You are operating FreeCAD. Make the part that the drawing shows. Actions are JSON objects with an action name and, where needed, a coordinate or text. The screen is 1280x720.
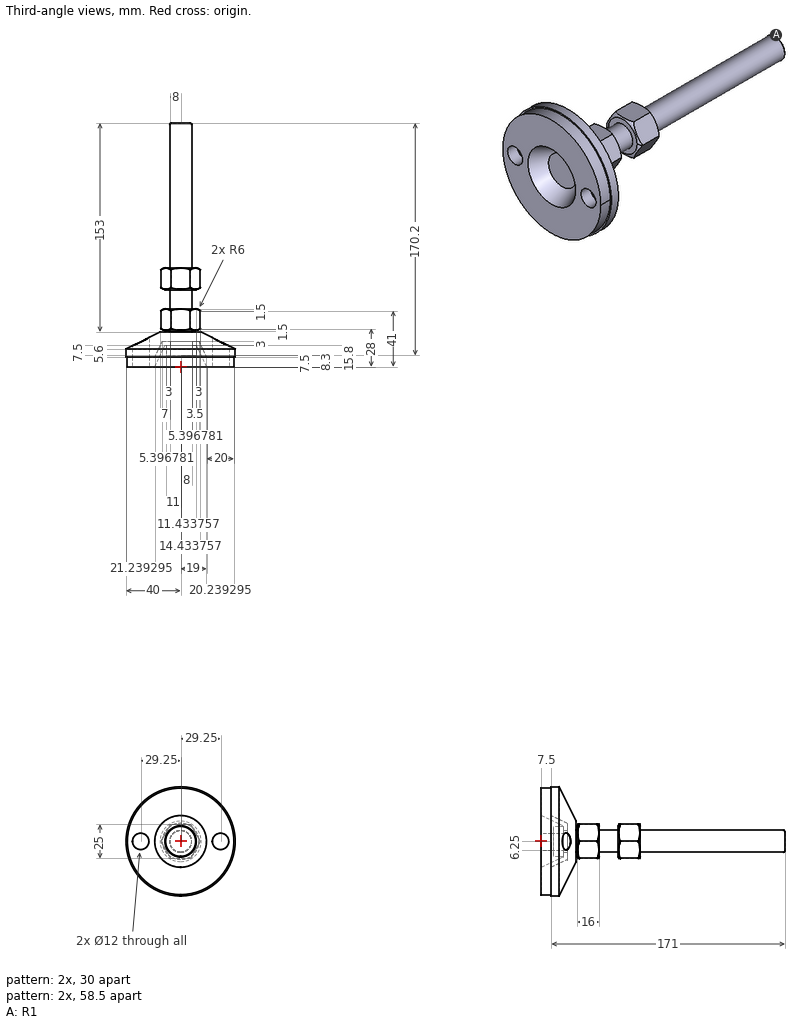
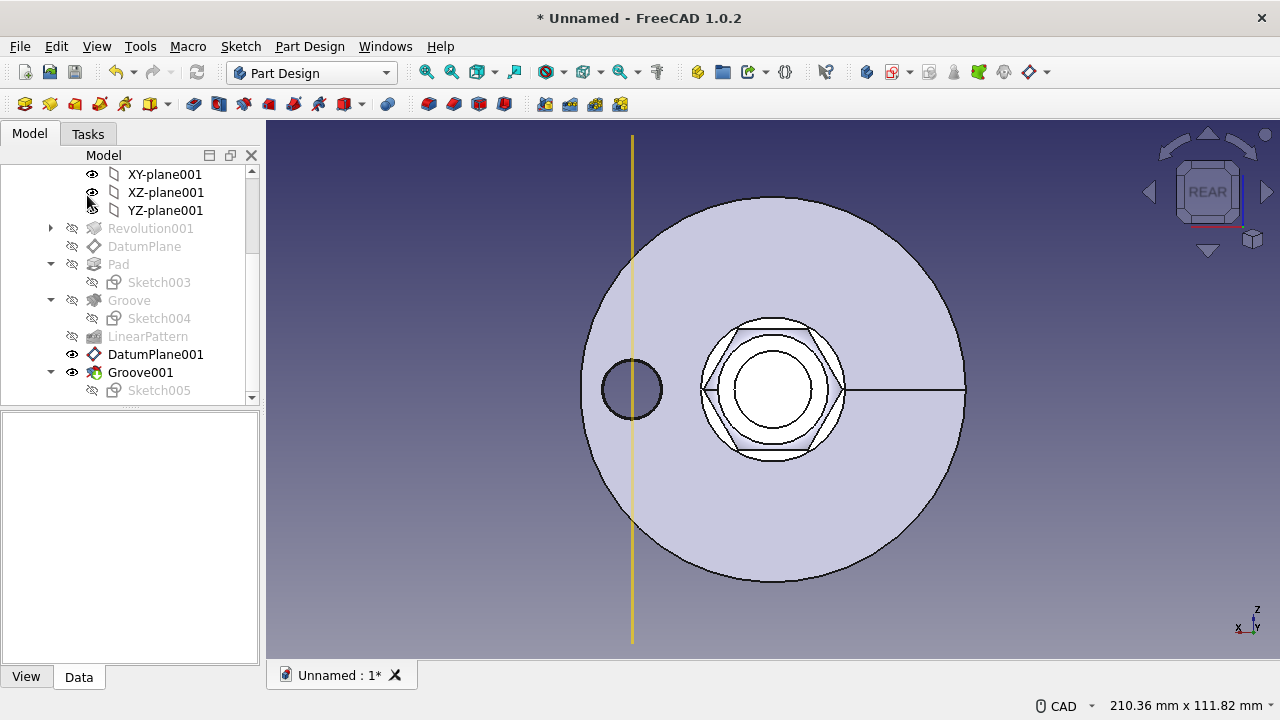
{"action": "left_click", "coordinate": [117, 354]}
{"action": "key", "text": "space"}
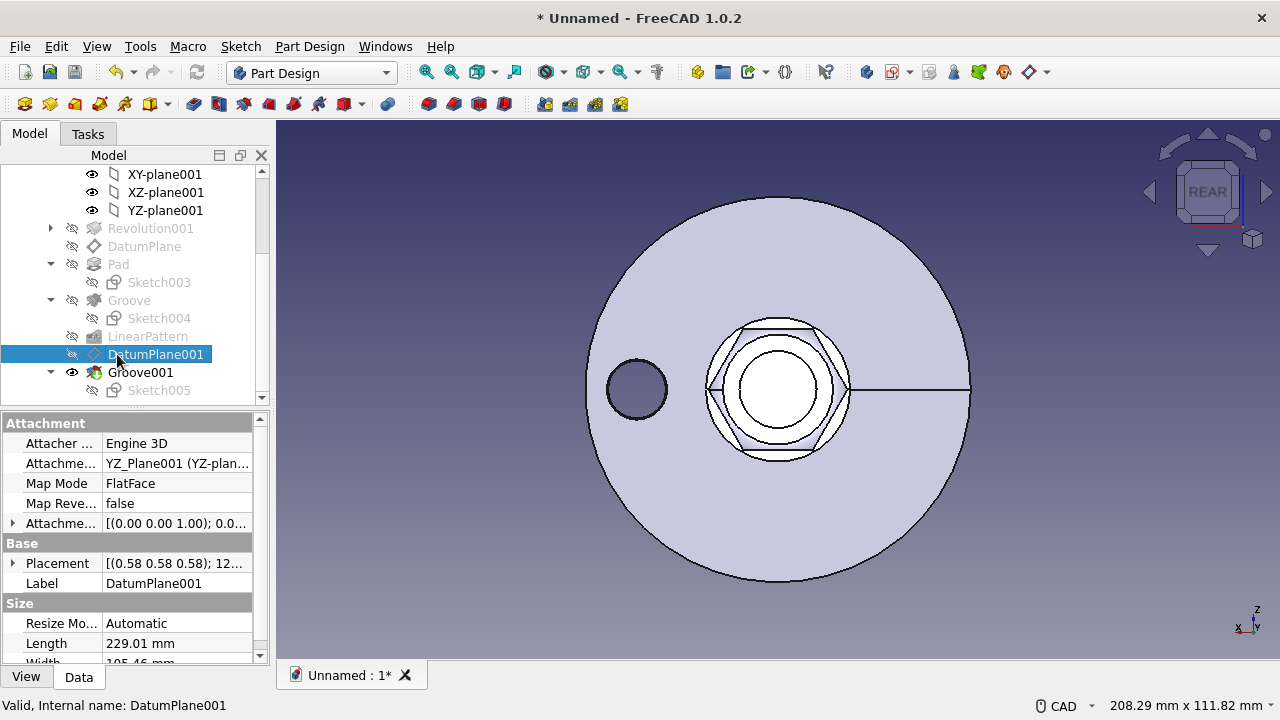
{"action": "left_click", "coordinate": [117, 372]}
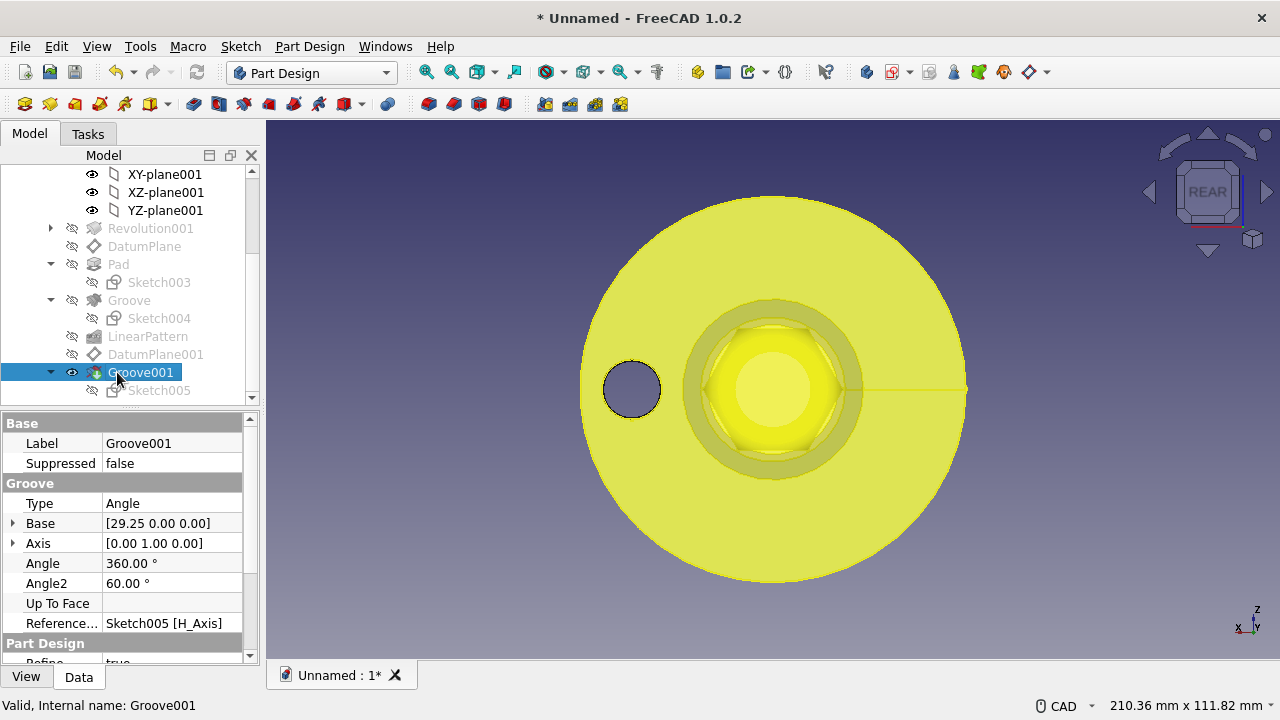
{"action": "left_click", "coordinate": [570, 104]}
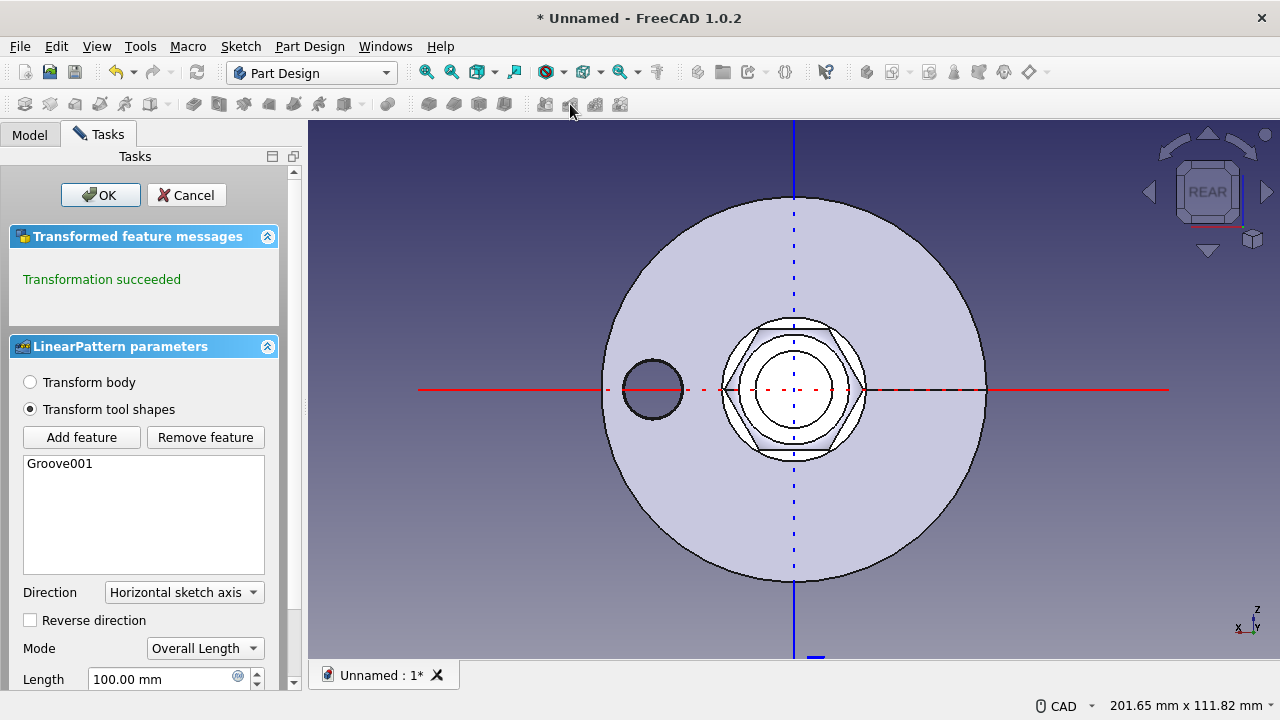
{"action": "left_click", "coordinate": [185, 592]}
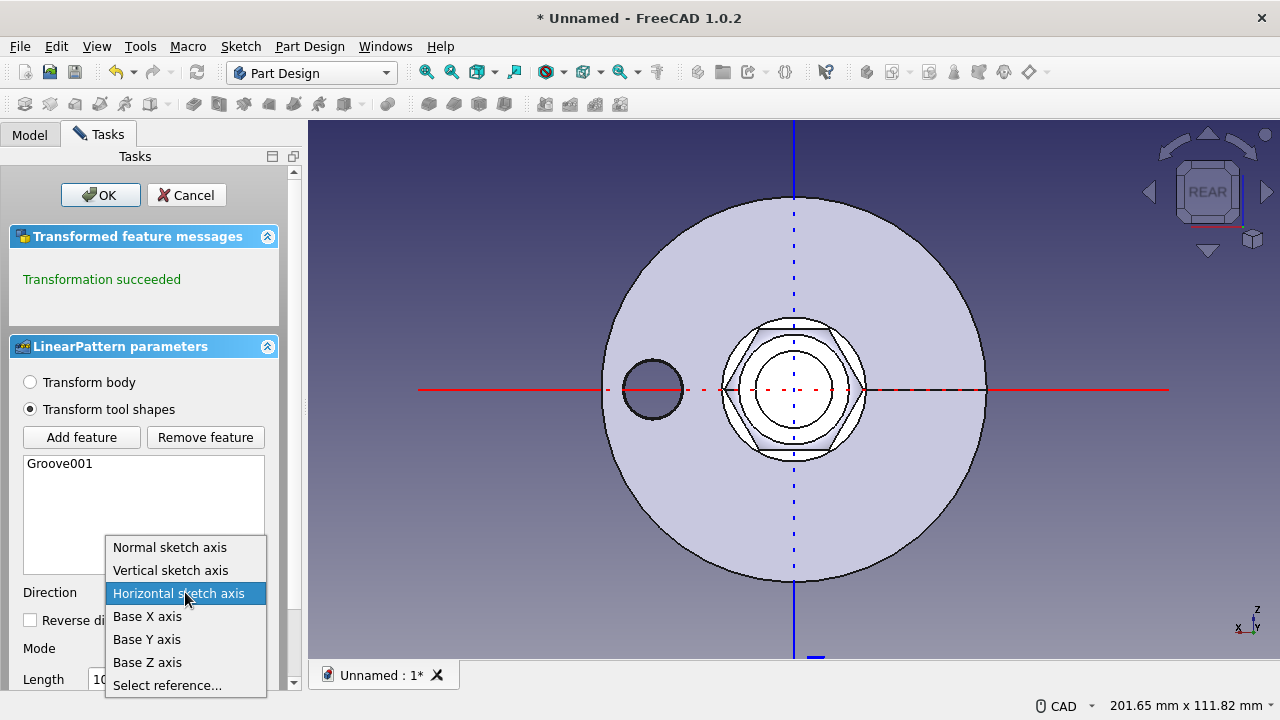
{"action": "left_click", "coordinate": [184, 616]}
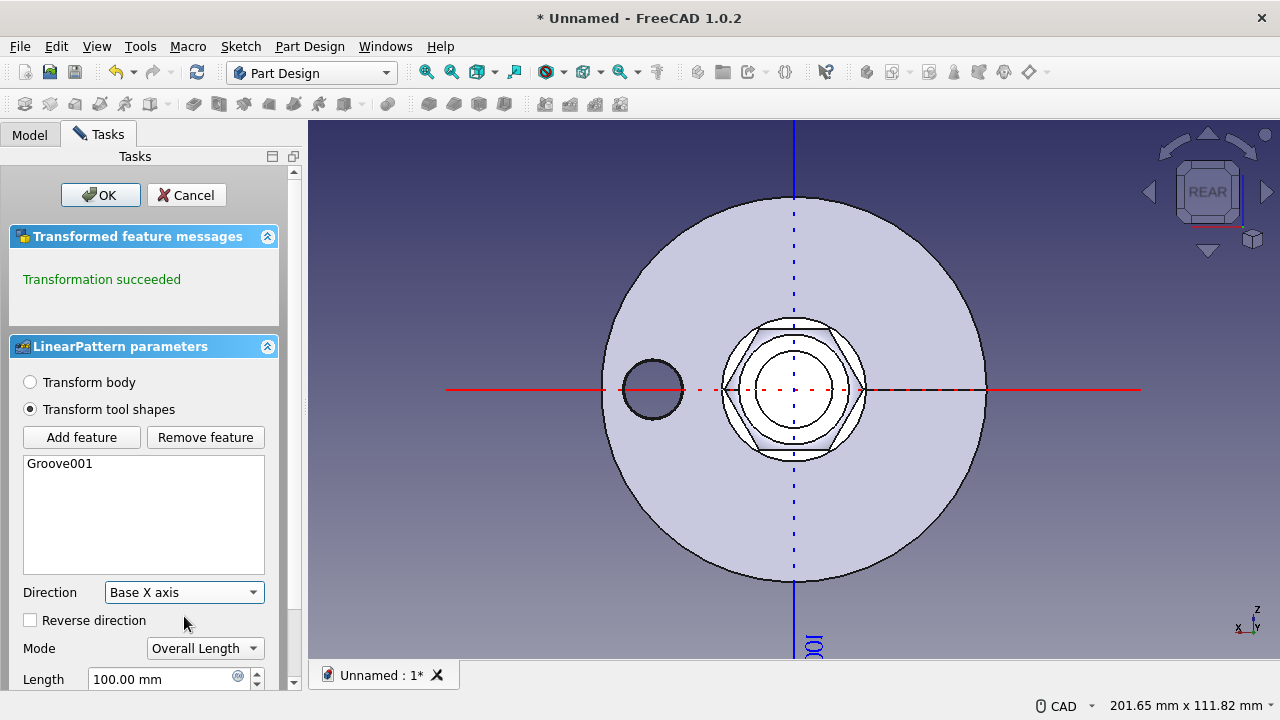
{"action": "left_click", "coordinate": [206, 648]}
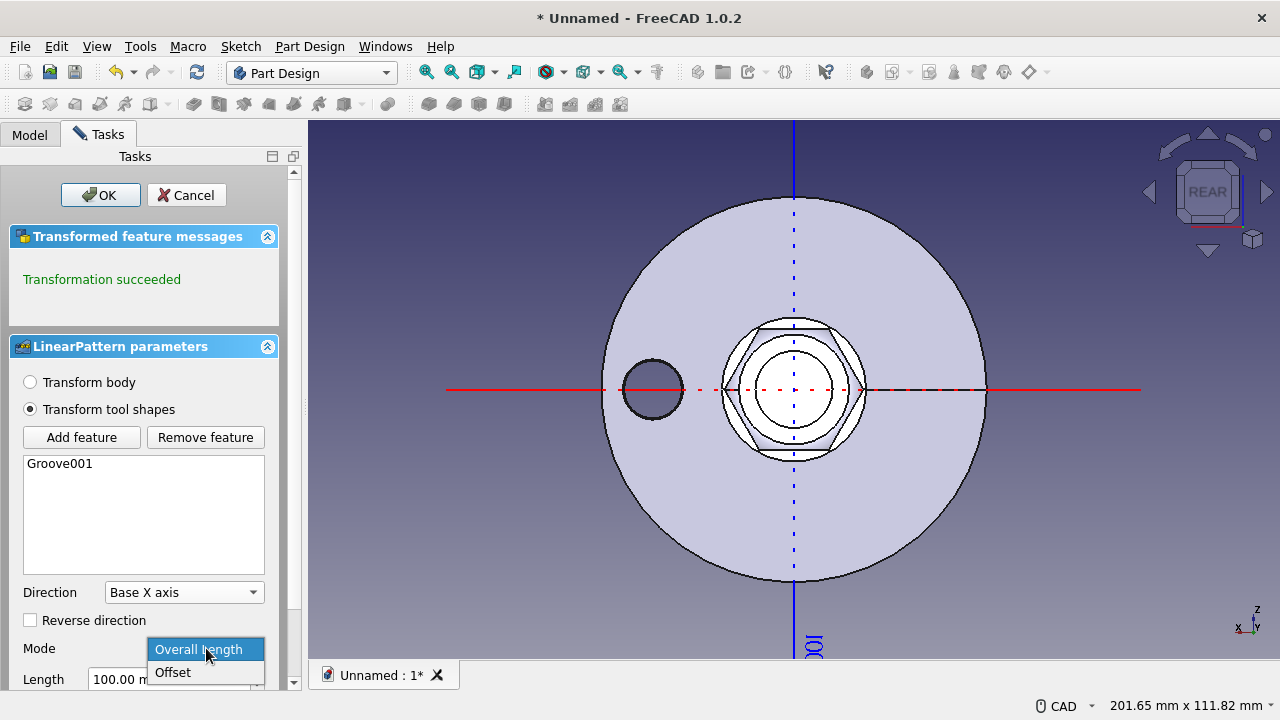
{"action": "left_click", "coordinate": [204, 672]}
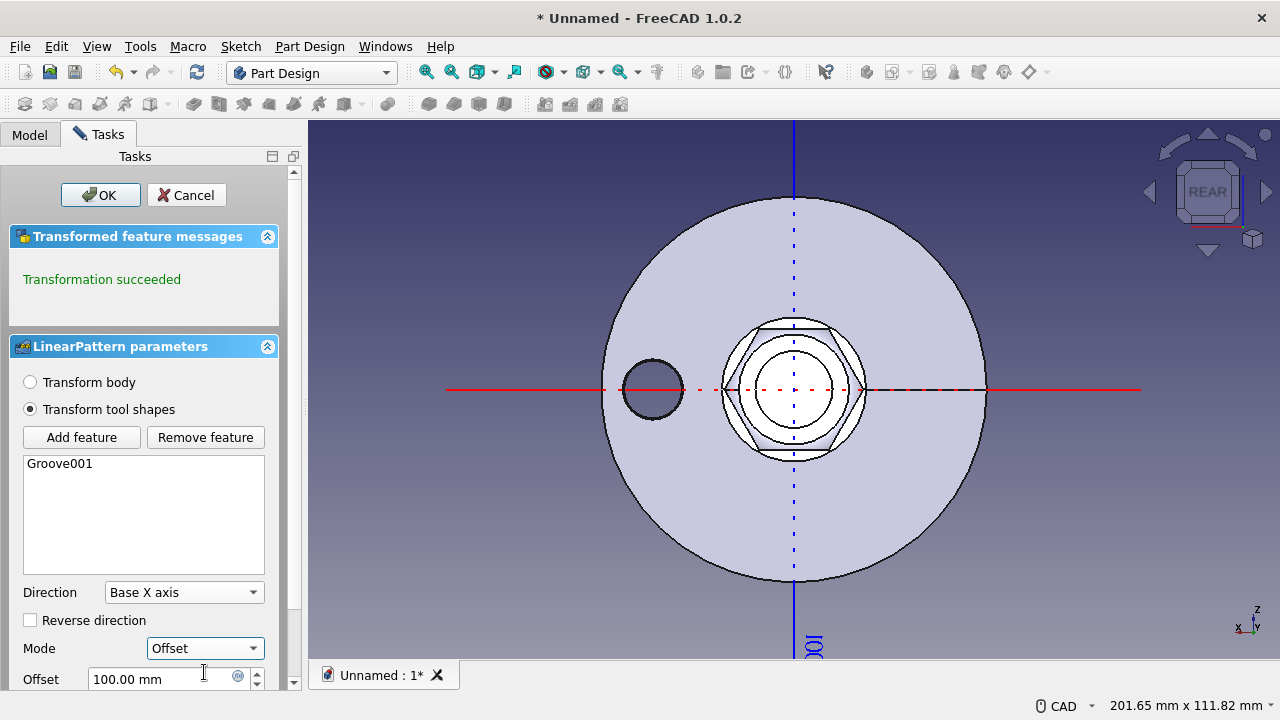
{"action": "scroll", "coordinate": [294, 428], "scroll_direction": "down", "scroll_amount": 2}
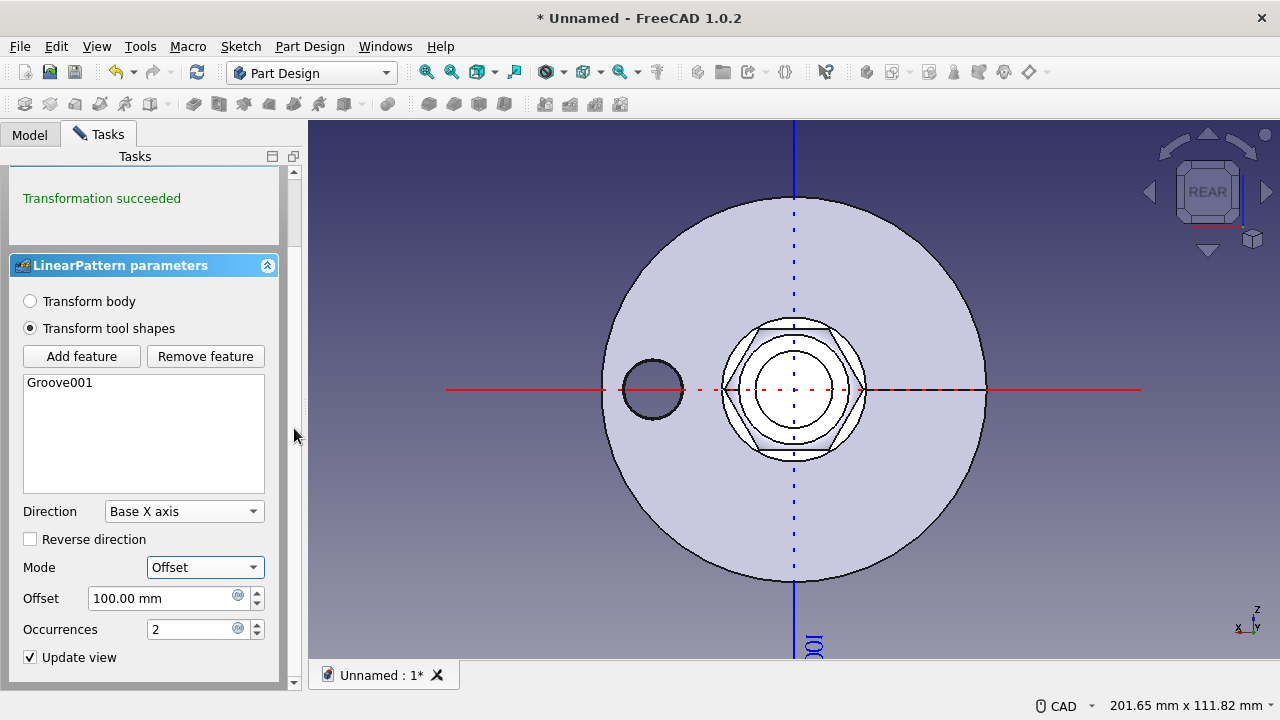
{"action": "triple_click", "coordinate": [170, 598]}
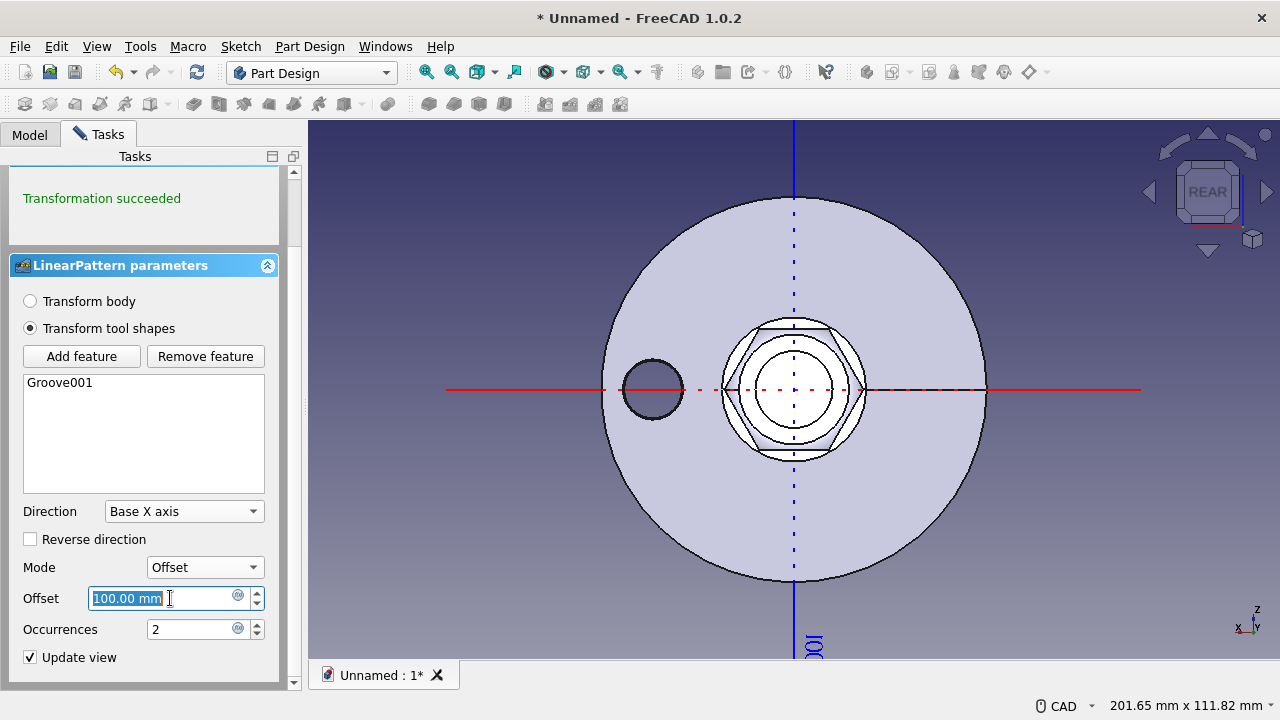
{"action": "type", "text": "58.5"}
{"action": "key", "text": "Tab"}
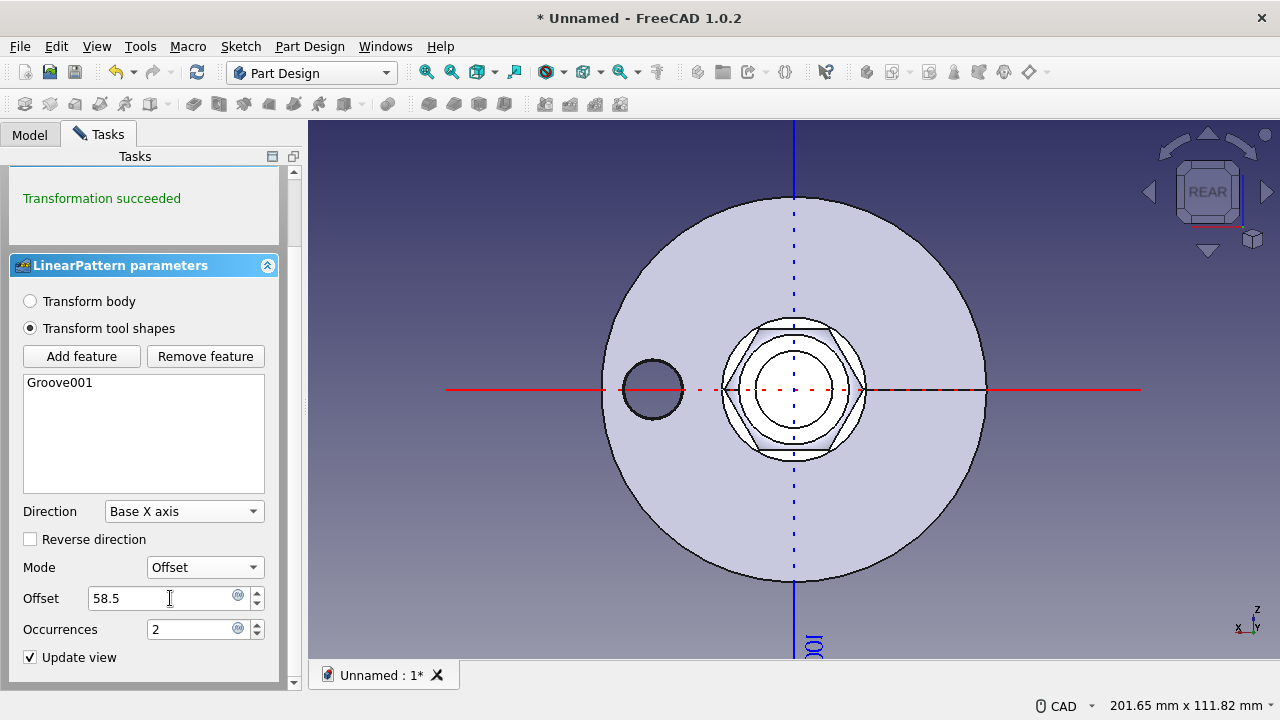
{"action": "triple_click", "coordinate": [199, 630]}